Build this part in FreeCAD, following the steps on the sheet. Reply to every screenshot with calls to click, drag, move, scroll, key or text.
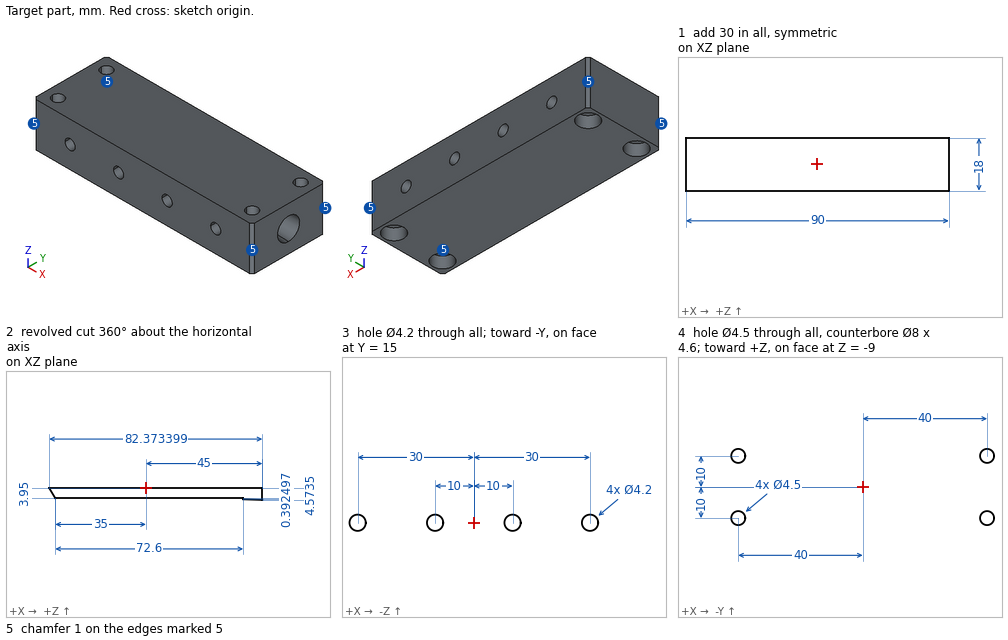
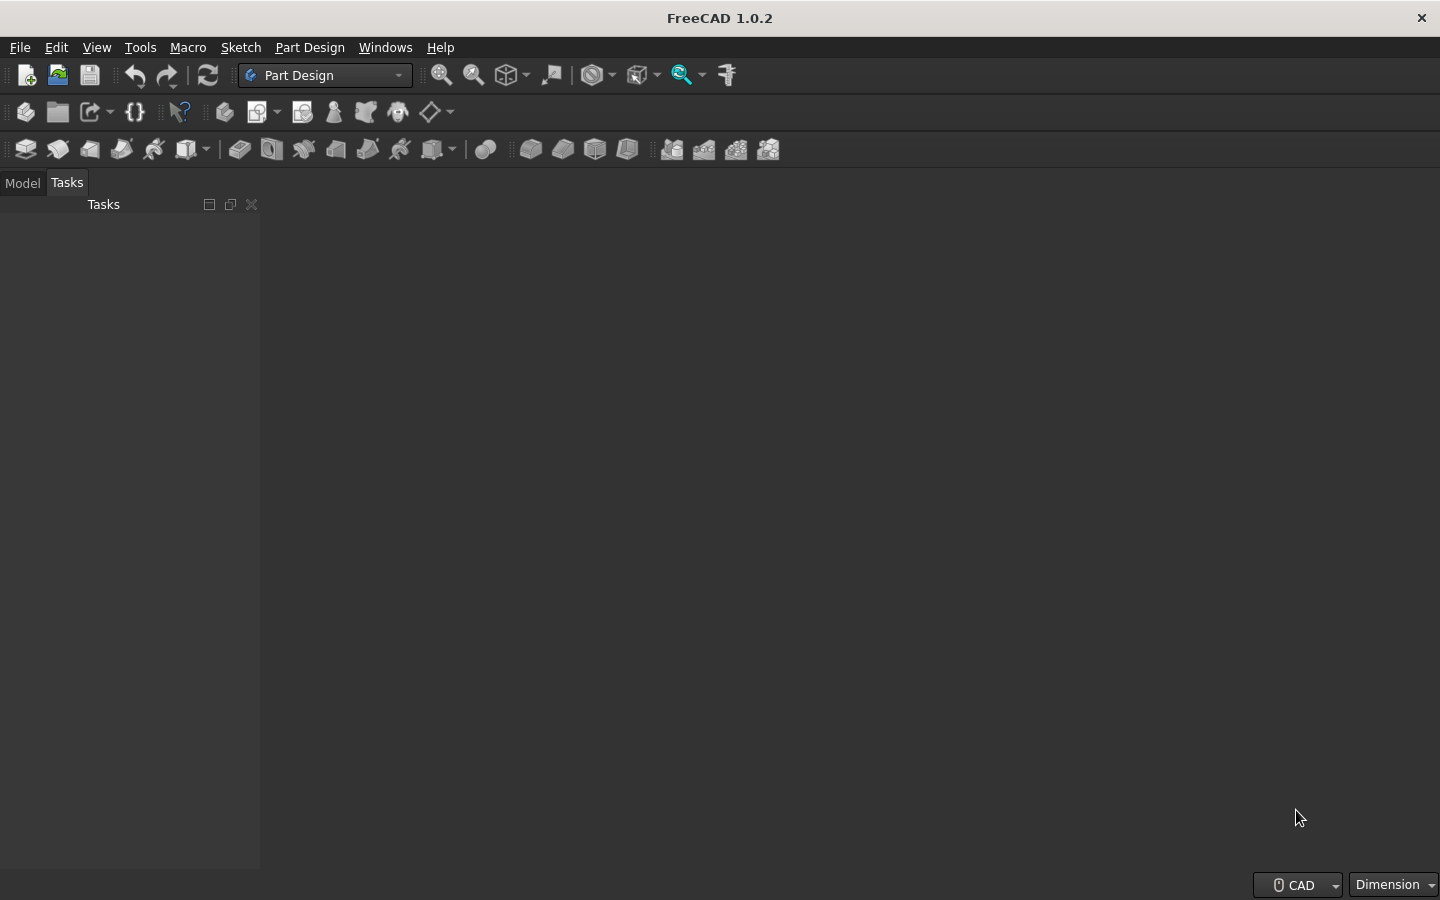
click(26, 76)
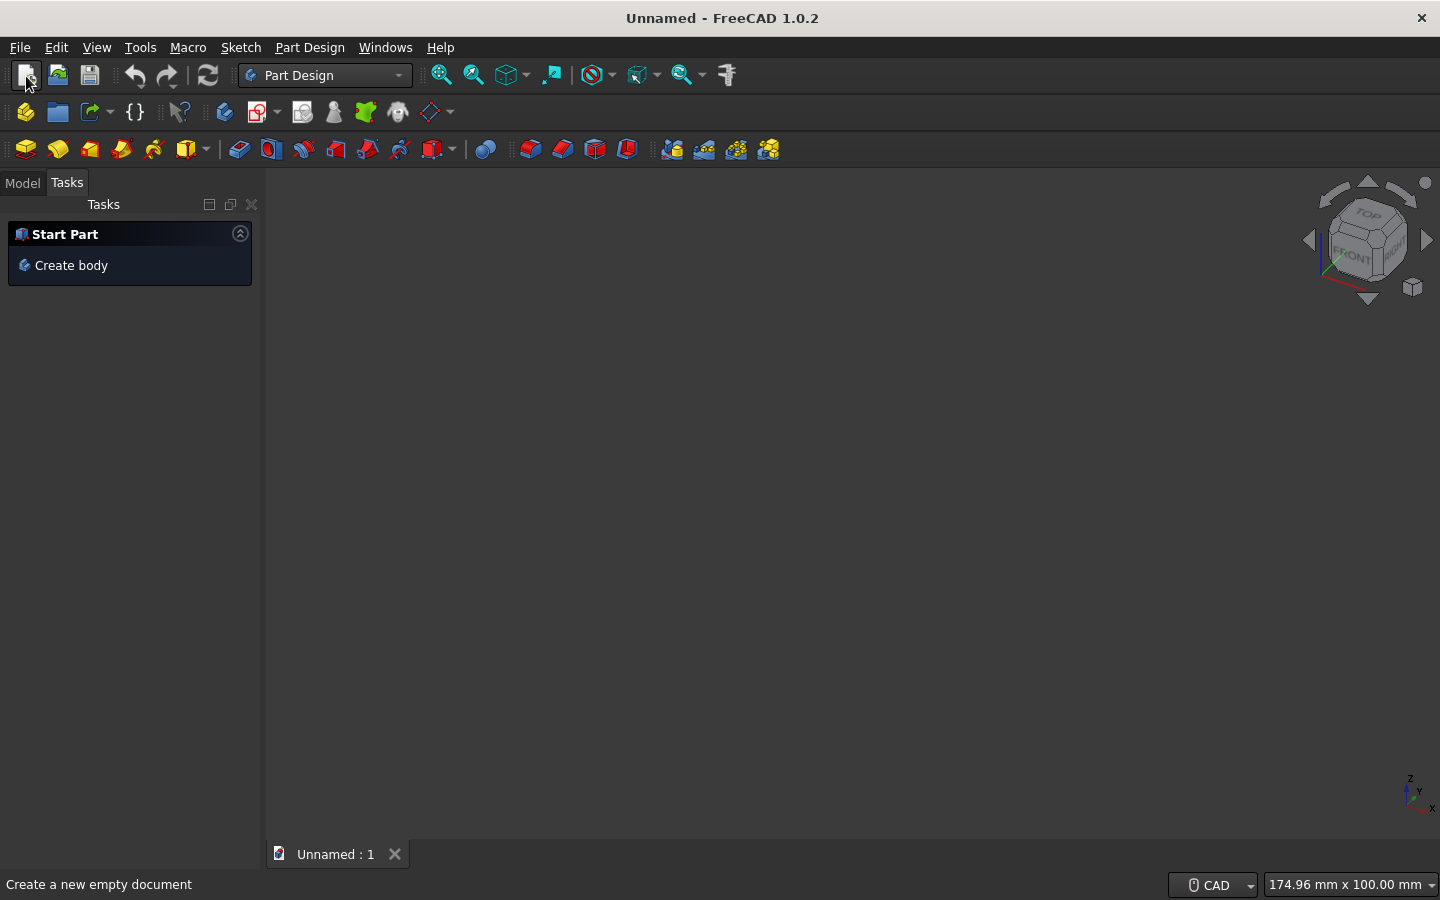
click(258, 112)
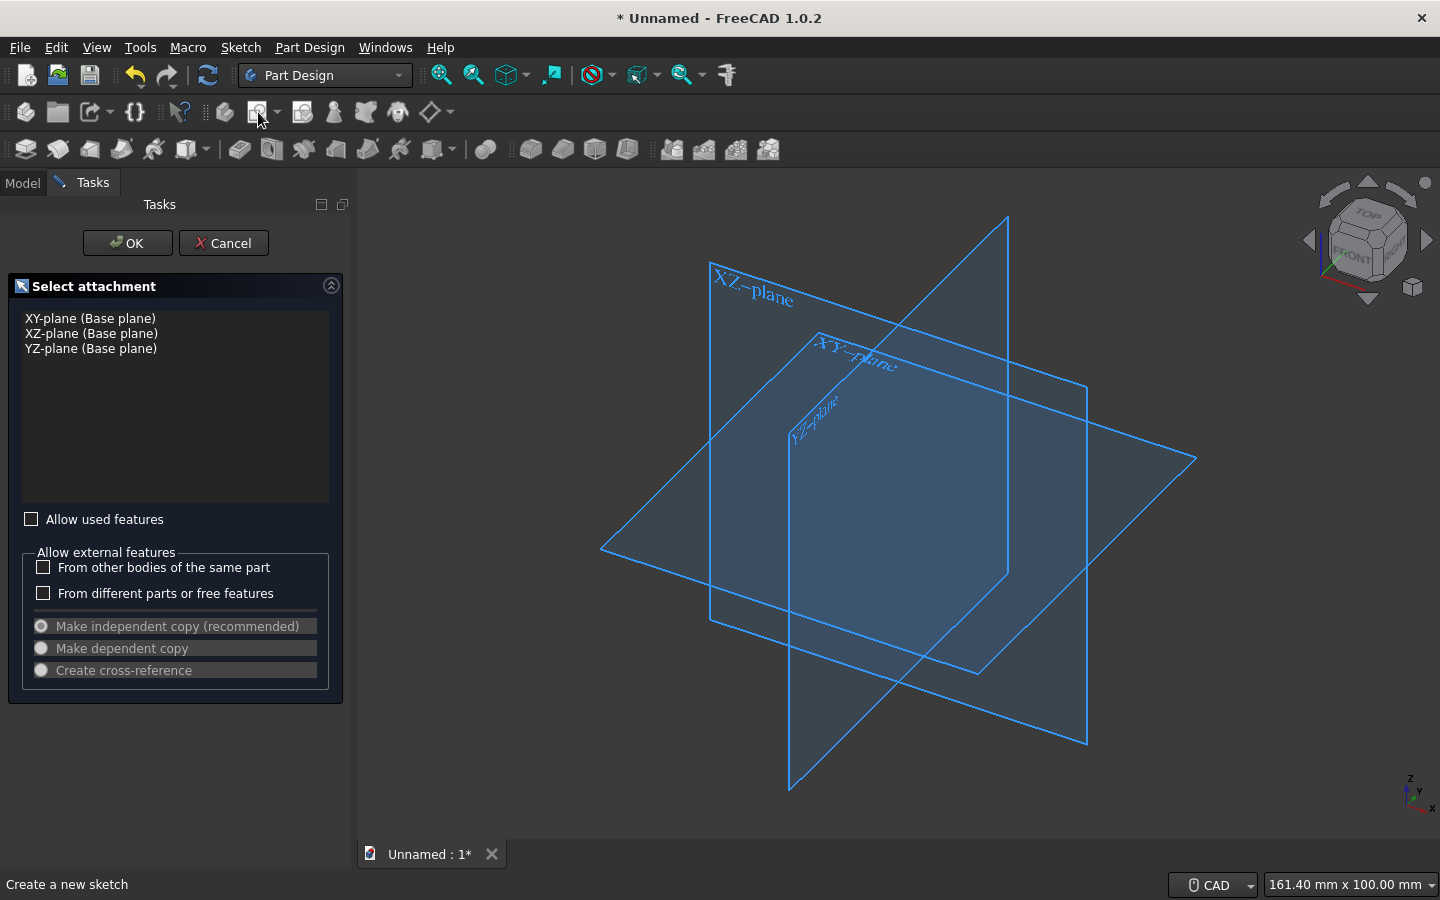
click(82, 334)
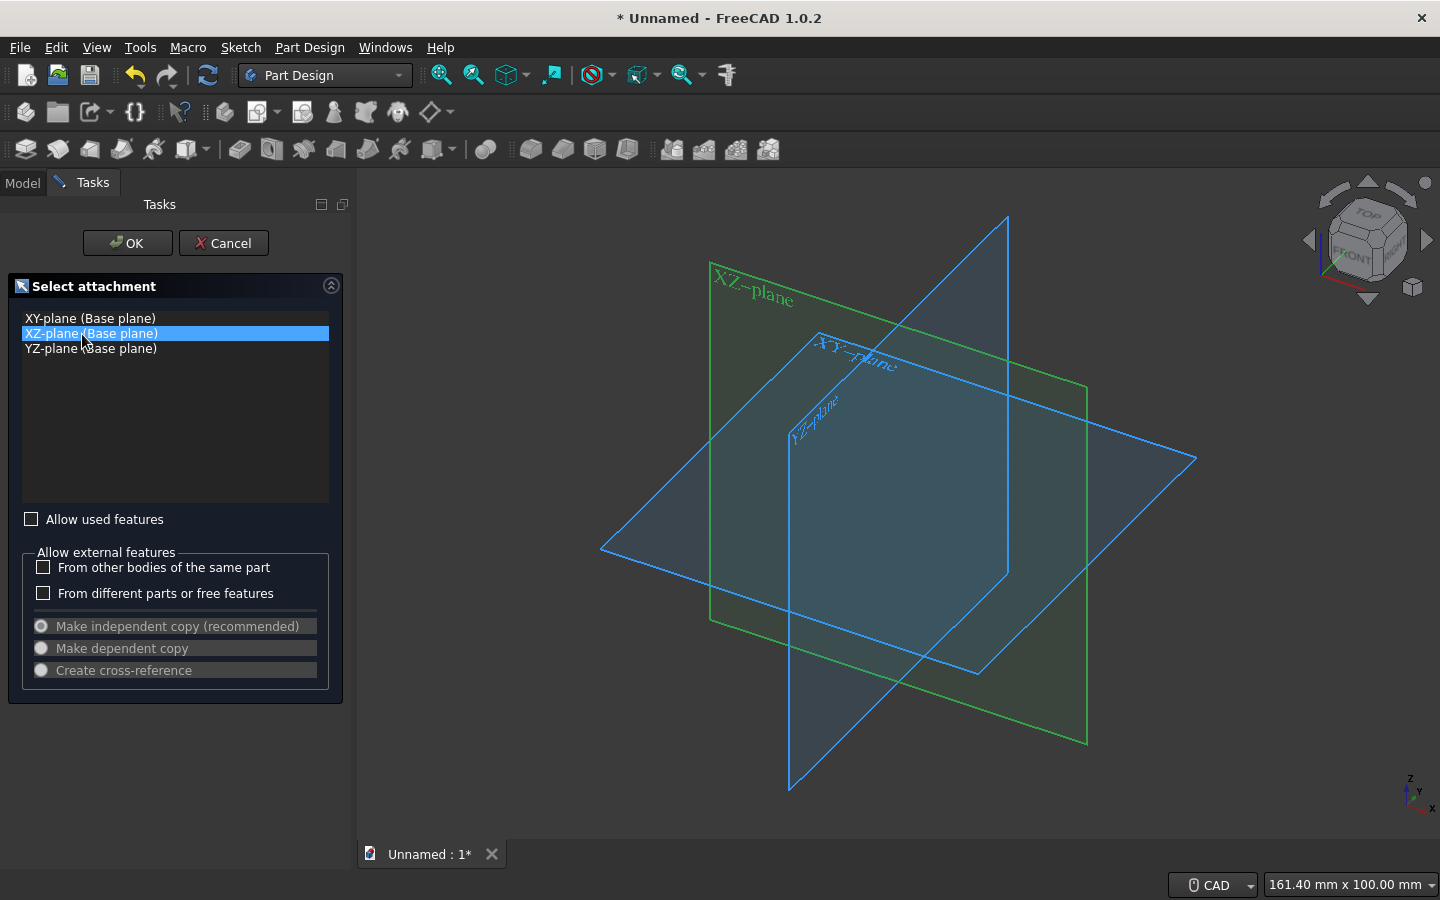
click(128, 243)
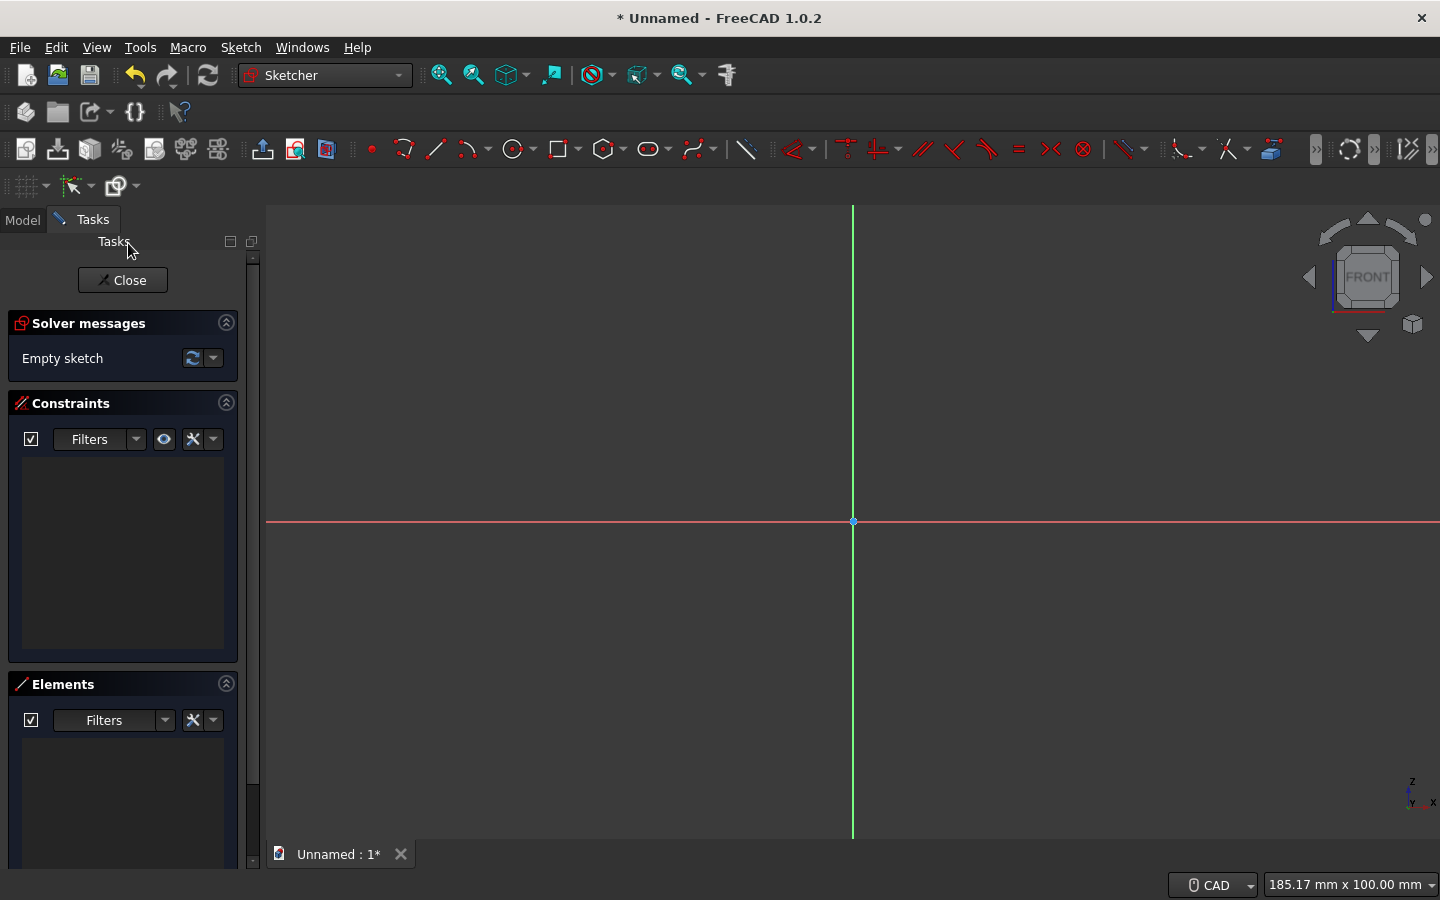
click(580, 150)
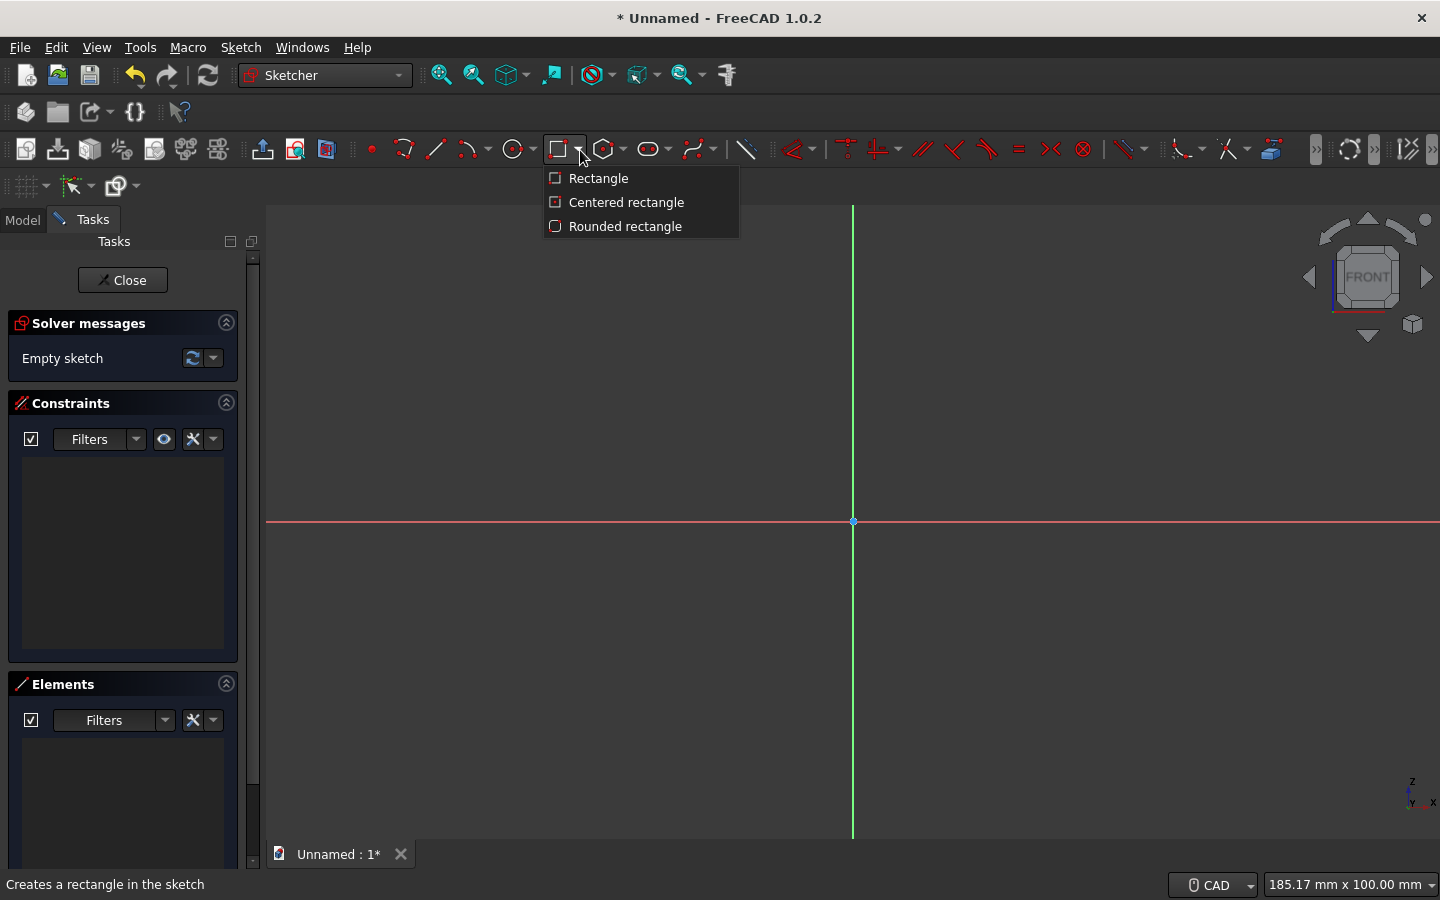
click(642, 202)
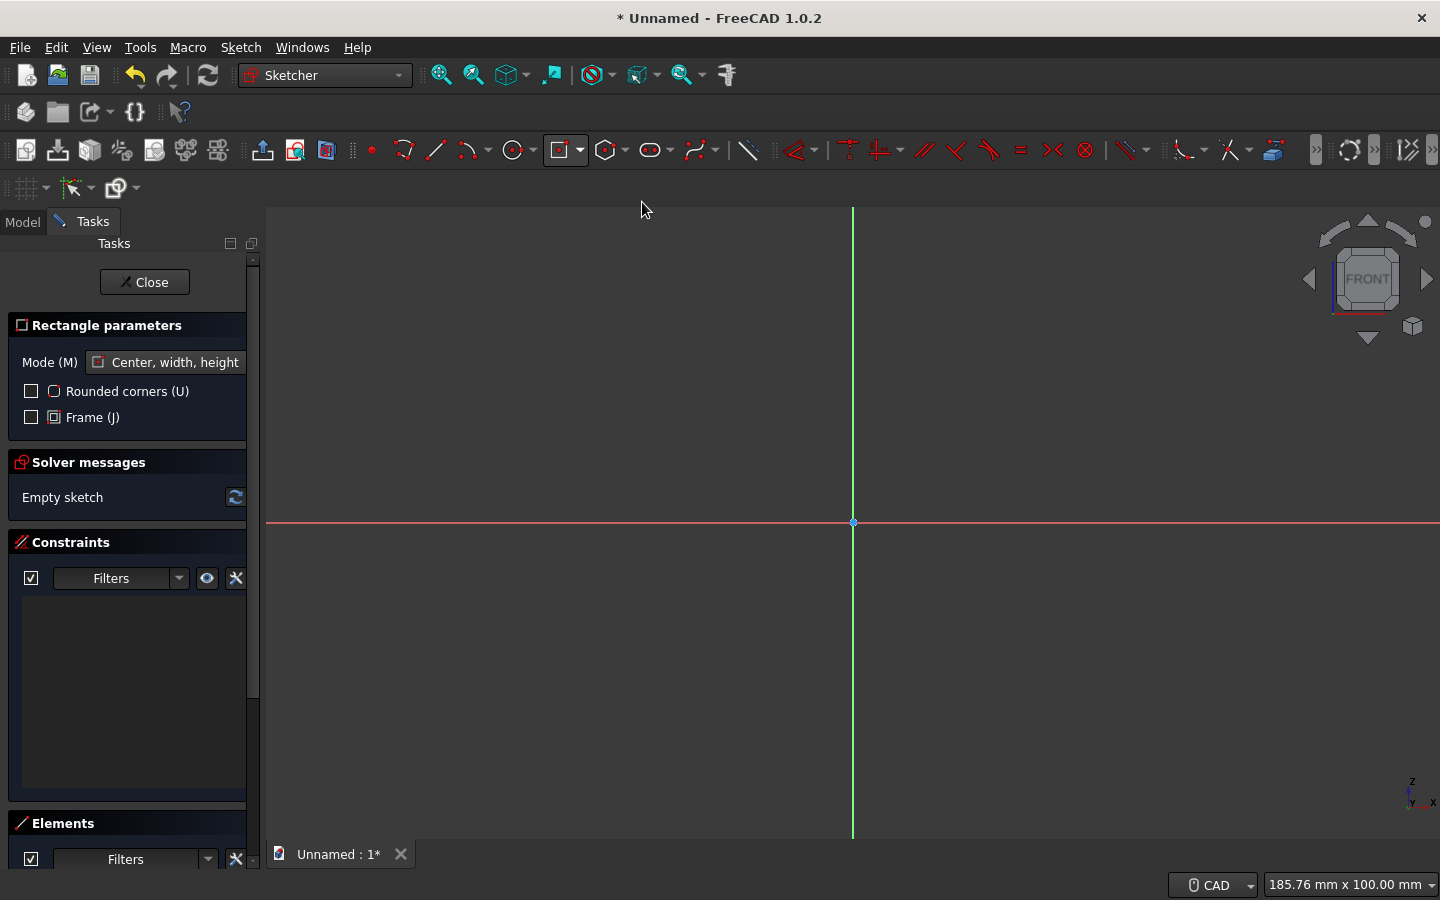
click(853, 523)
click(1137, 466)
key(Escape)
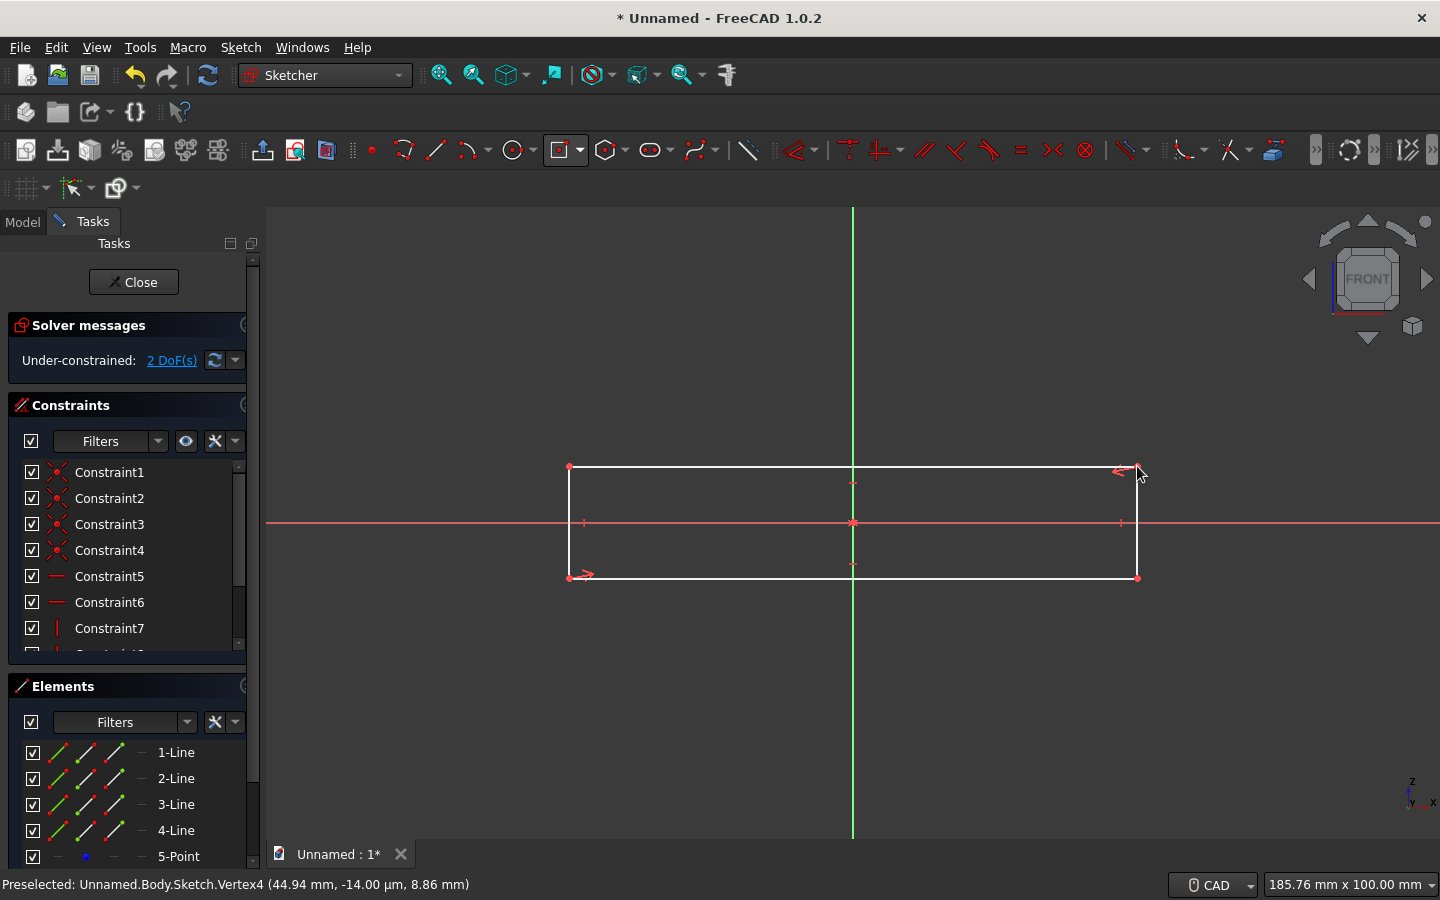
click(739, 579)